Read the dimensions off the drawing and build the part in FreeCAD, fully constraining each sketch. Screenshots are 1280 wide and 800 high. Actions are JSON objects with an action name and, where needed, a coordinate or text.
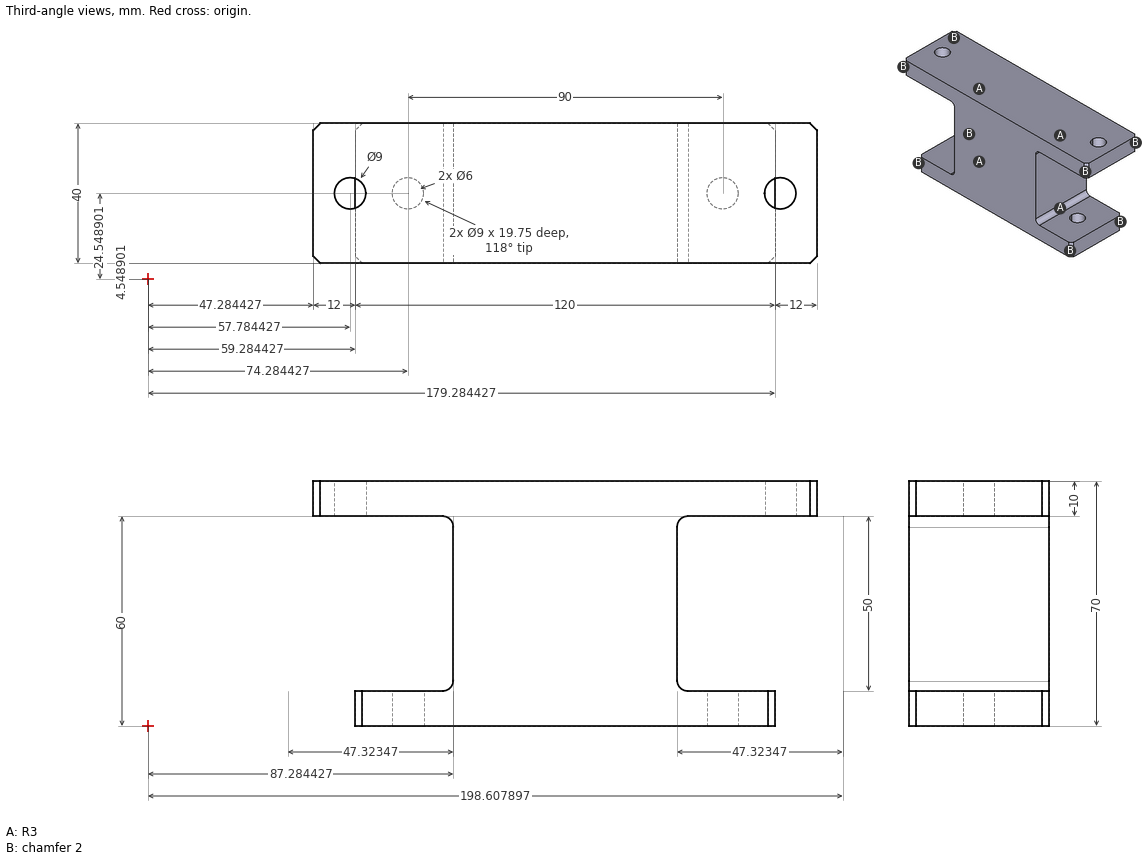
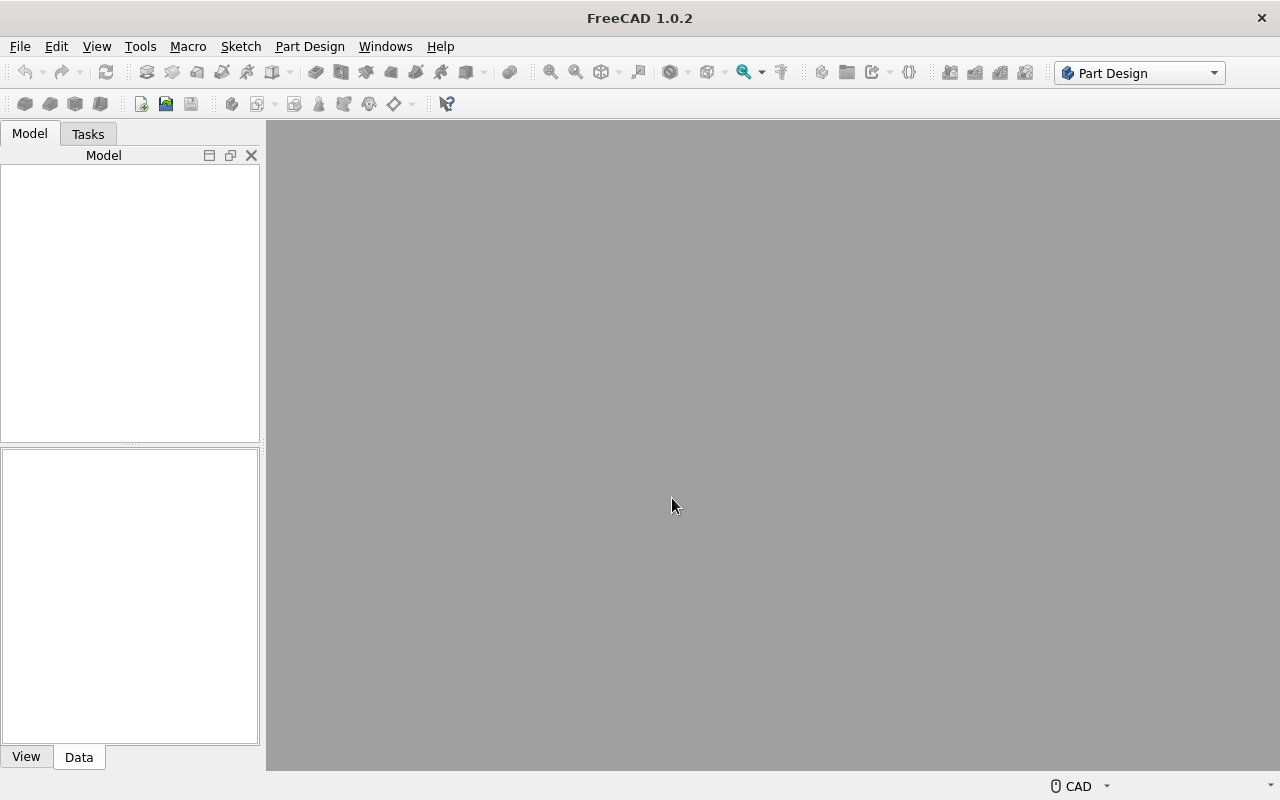
{"action": "key", "text": "ctrl+n"}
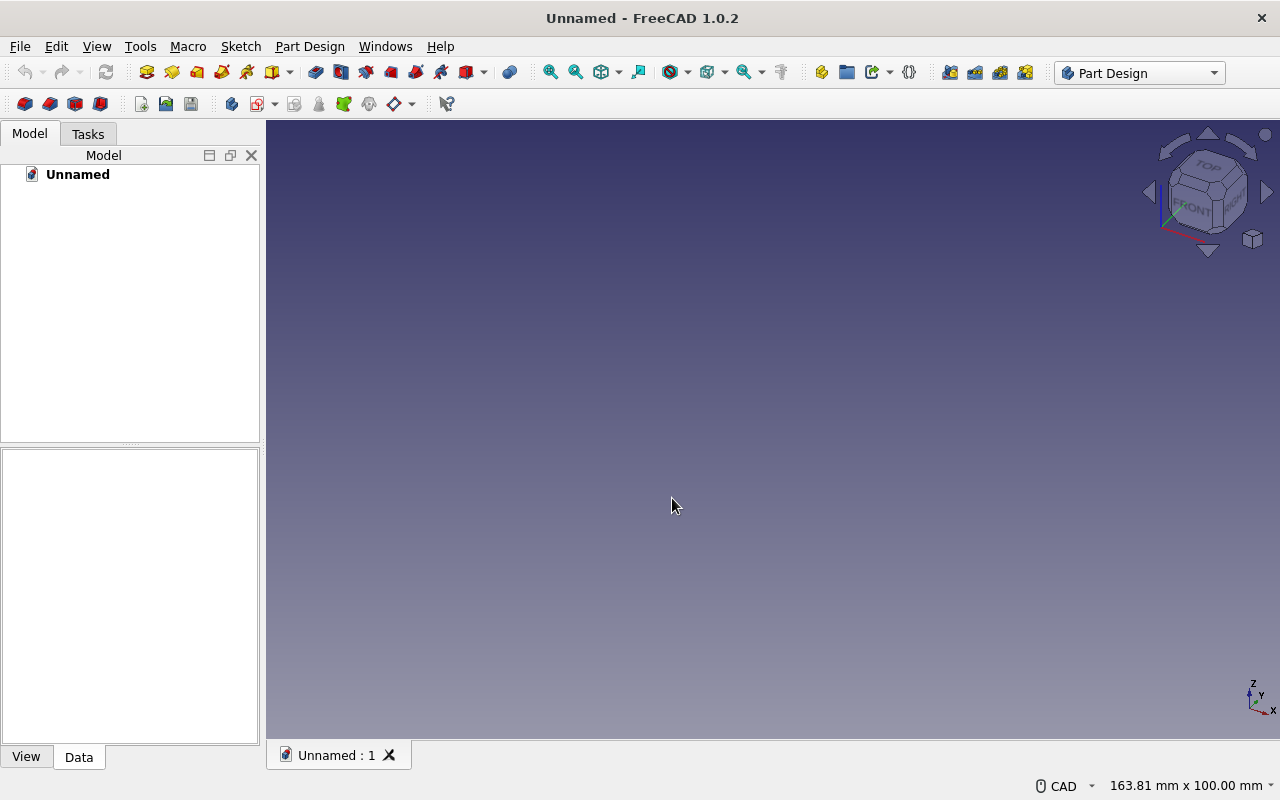
{"action": "left_click", "coordinate": [256, 104]}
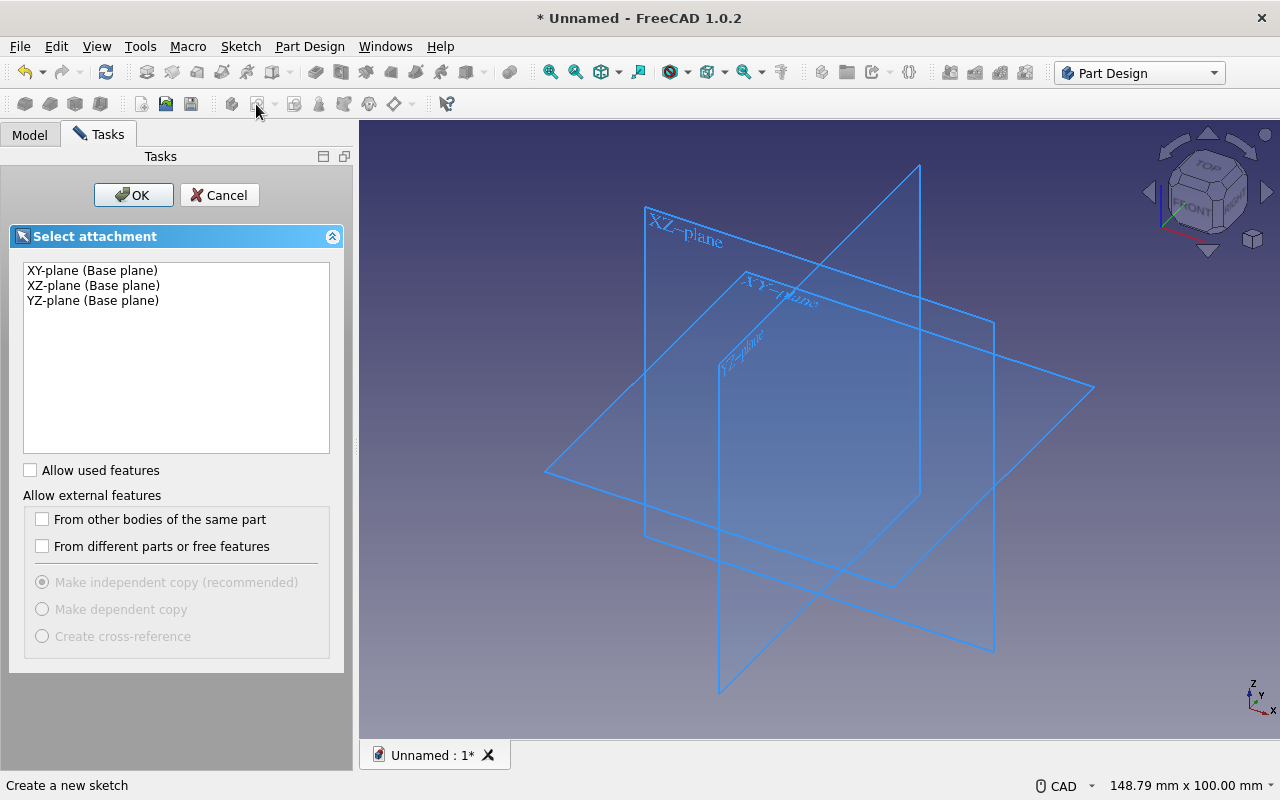
{"action": "left_click", "coordinate": [84, 270]}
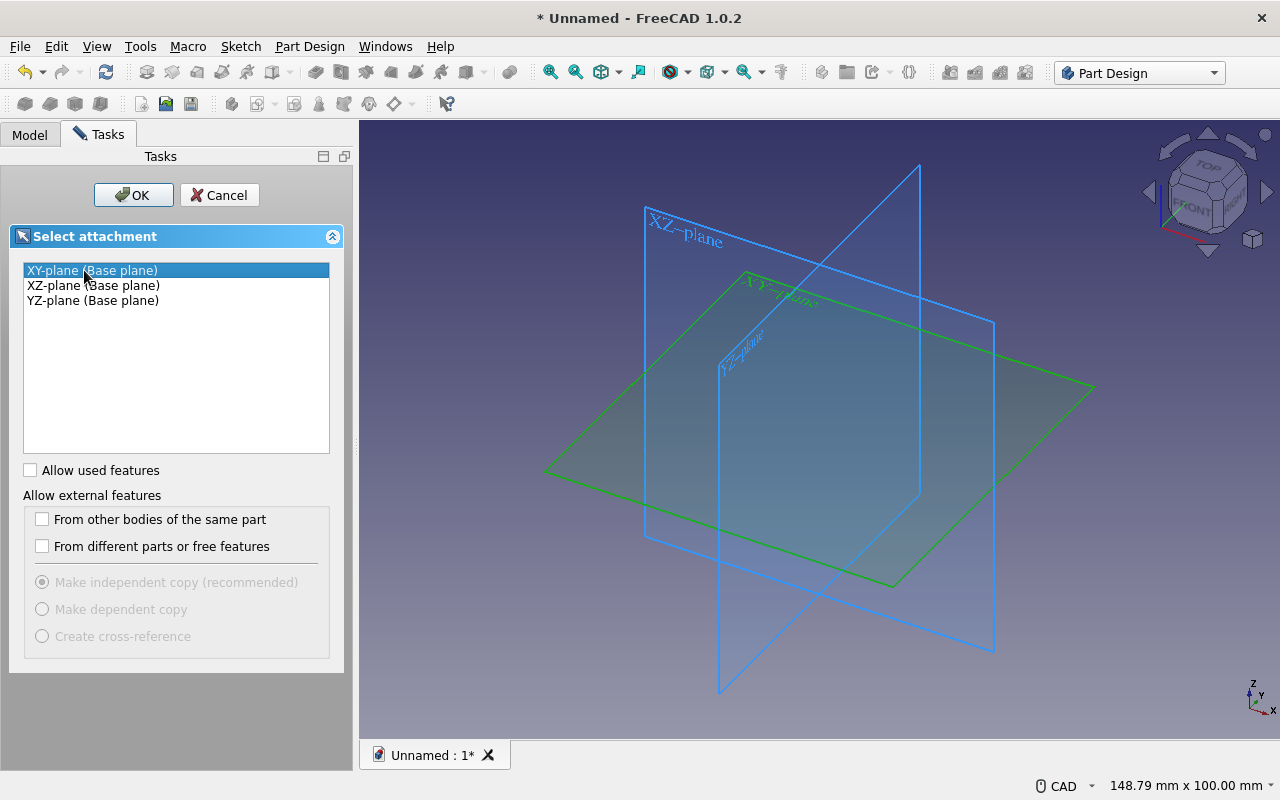
{"action": "left_click", "coordinate": [134, 195]}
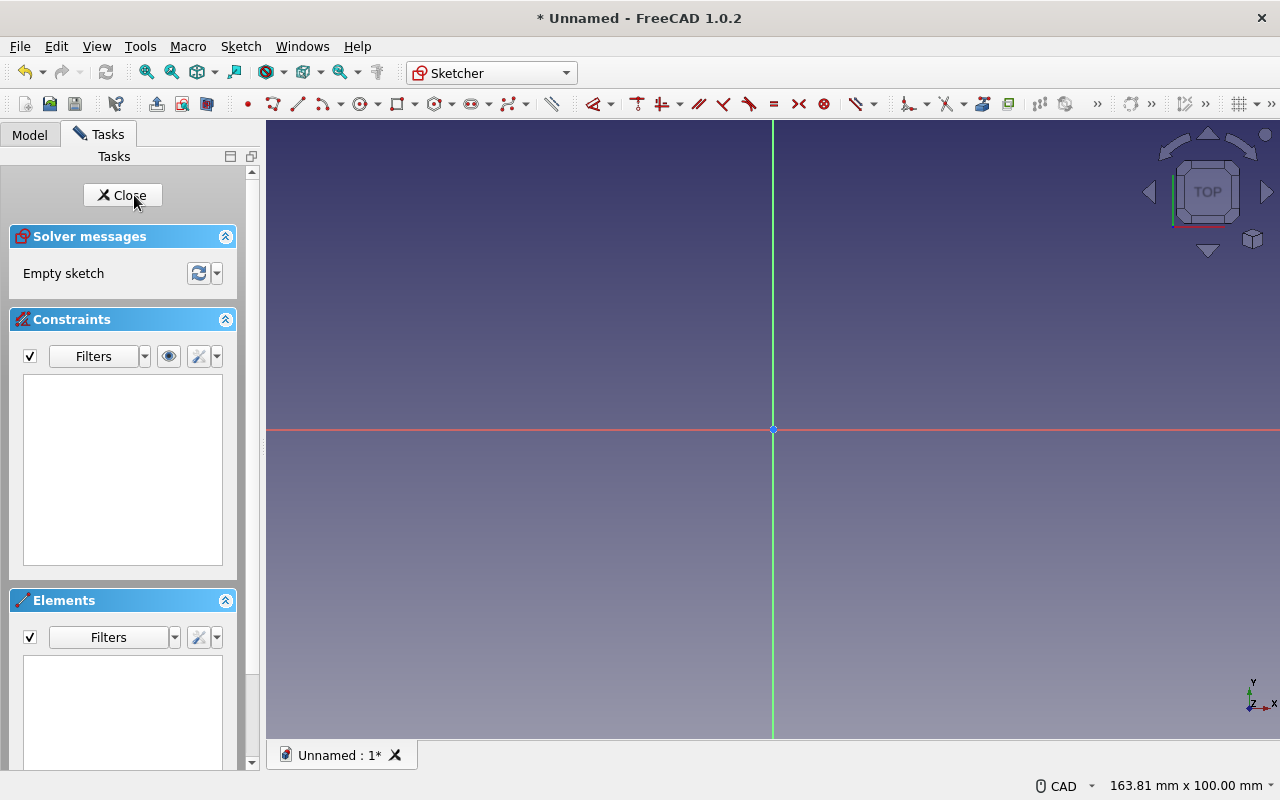
{"action": "scroll", "coordinate": [294, 542], "scroll_direction": "down", "scroll_amount": 4}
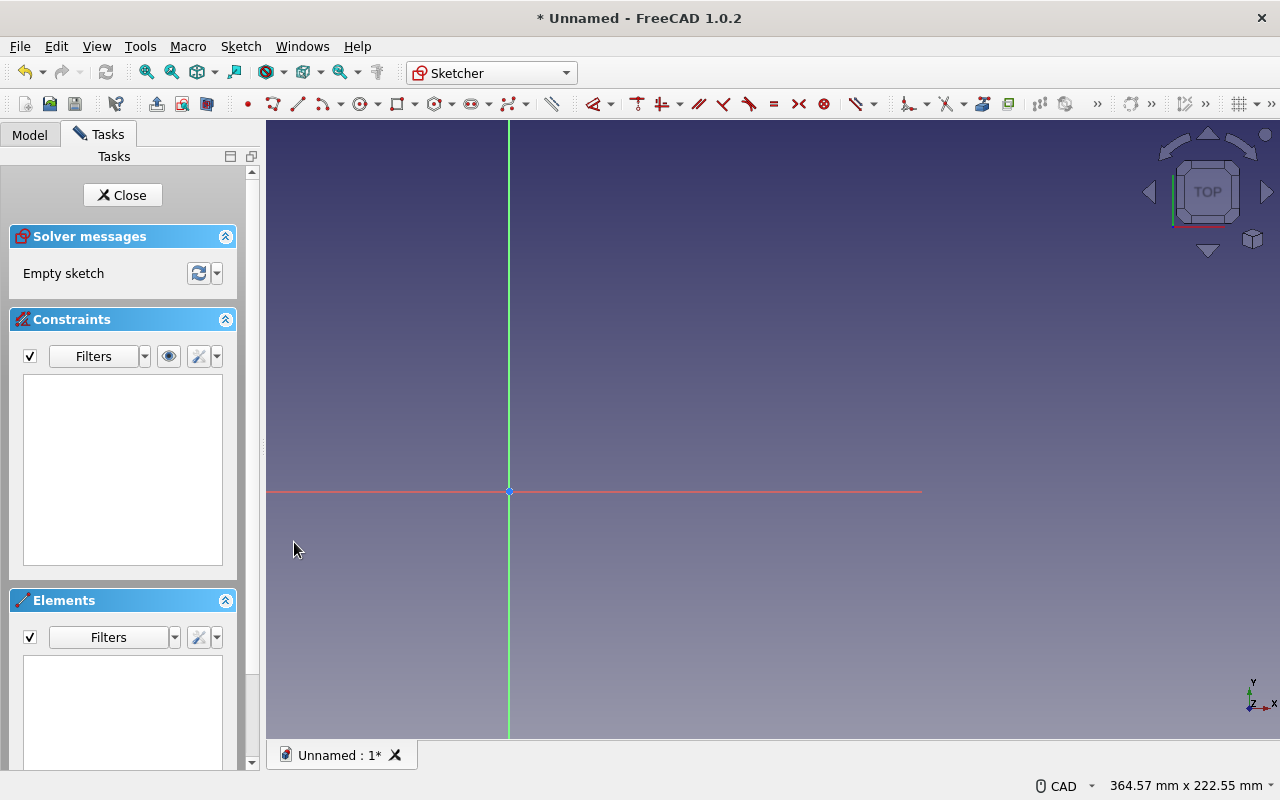
{"action": "key", "text": "g r"}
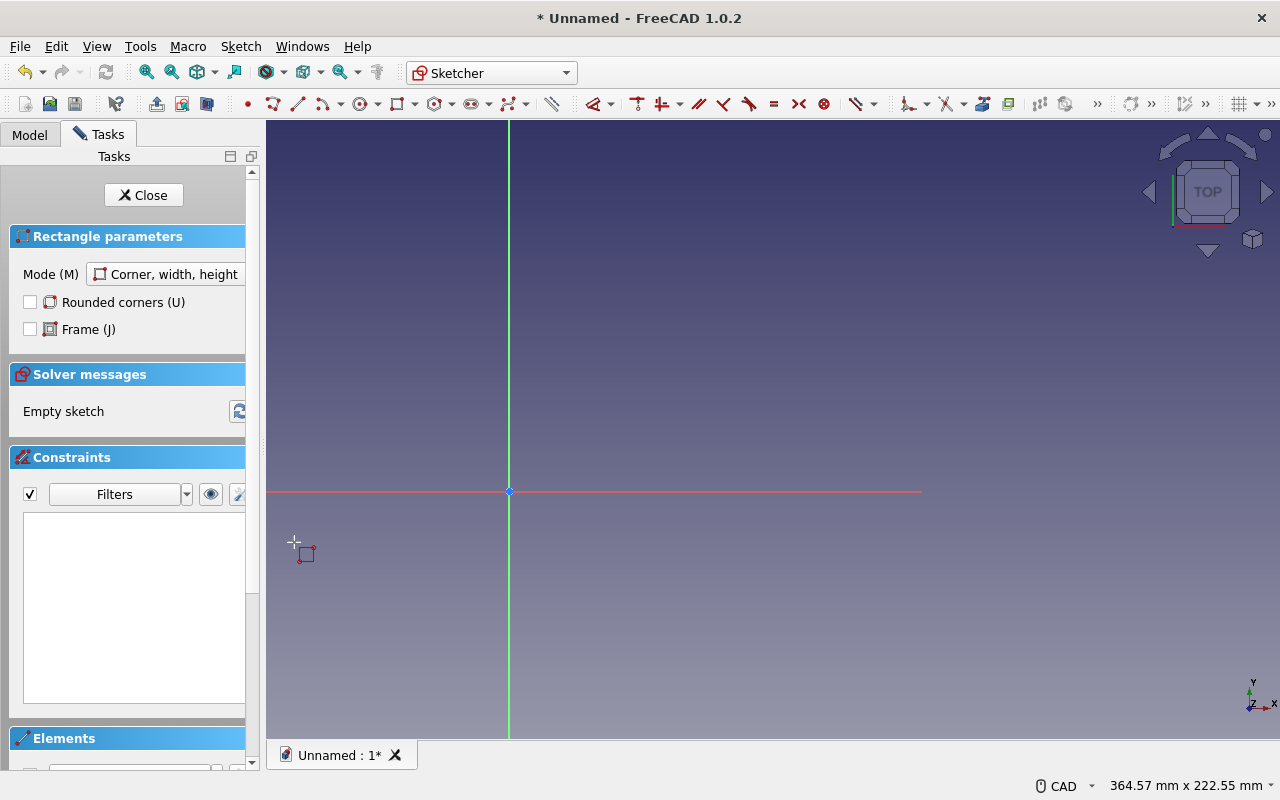
{"action": "left_click", "coordinate": [674, 368]}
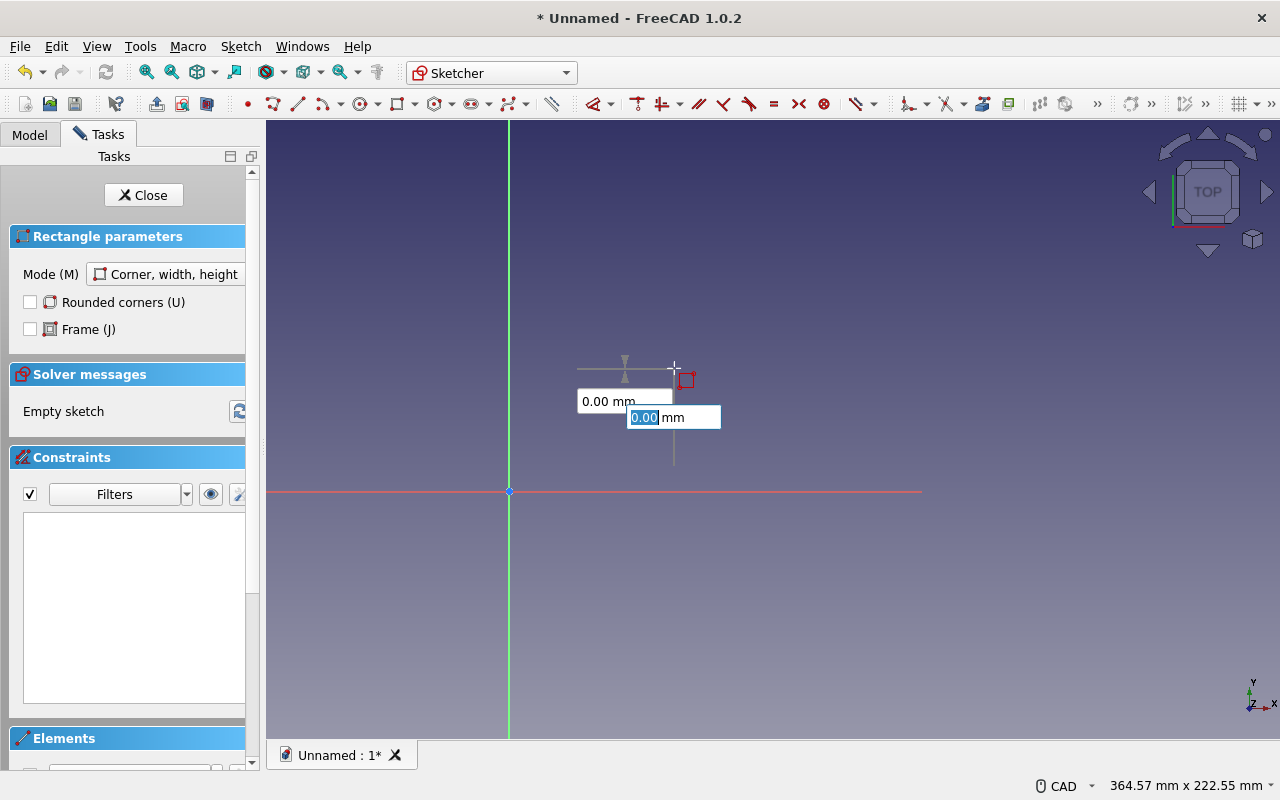
{"action": "scroll", "coordinate": [1008, 479], "scroll_direction": "up", "scroll_amount": 2}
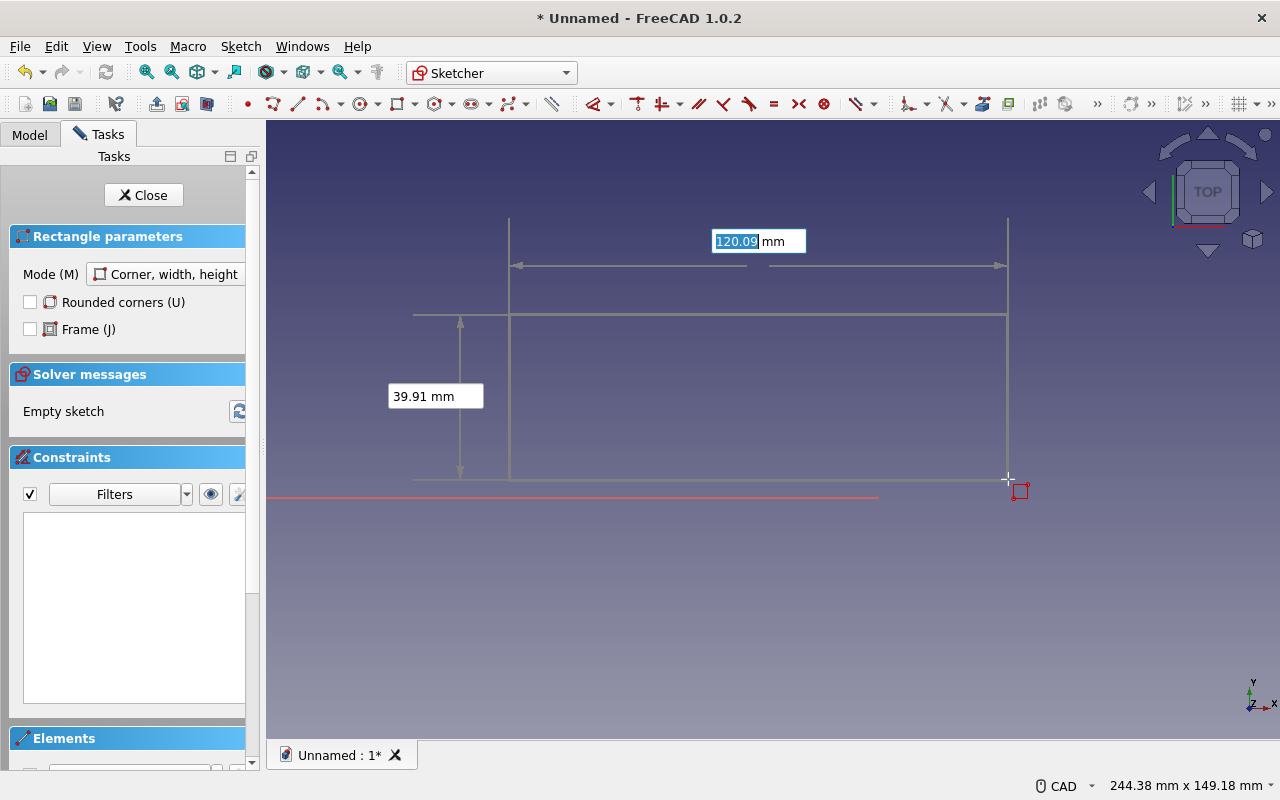
{"action": "left_click", "coordinate": [1007, 479]}
{"action": "key", "text": "Escape"}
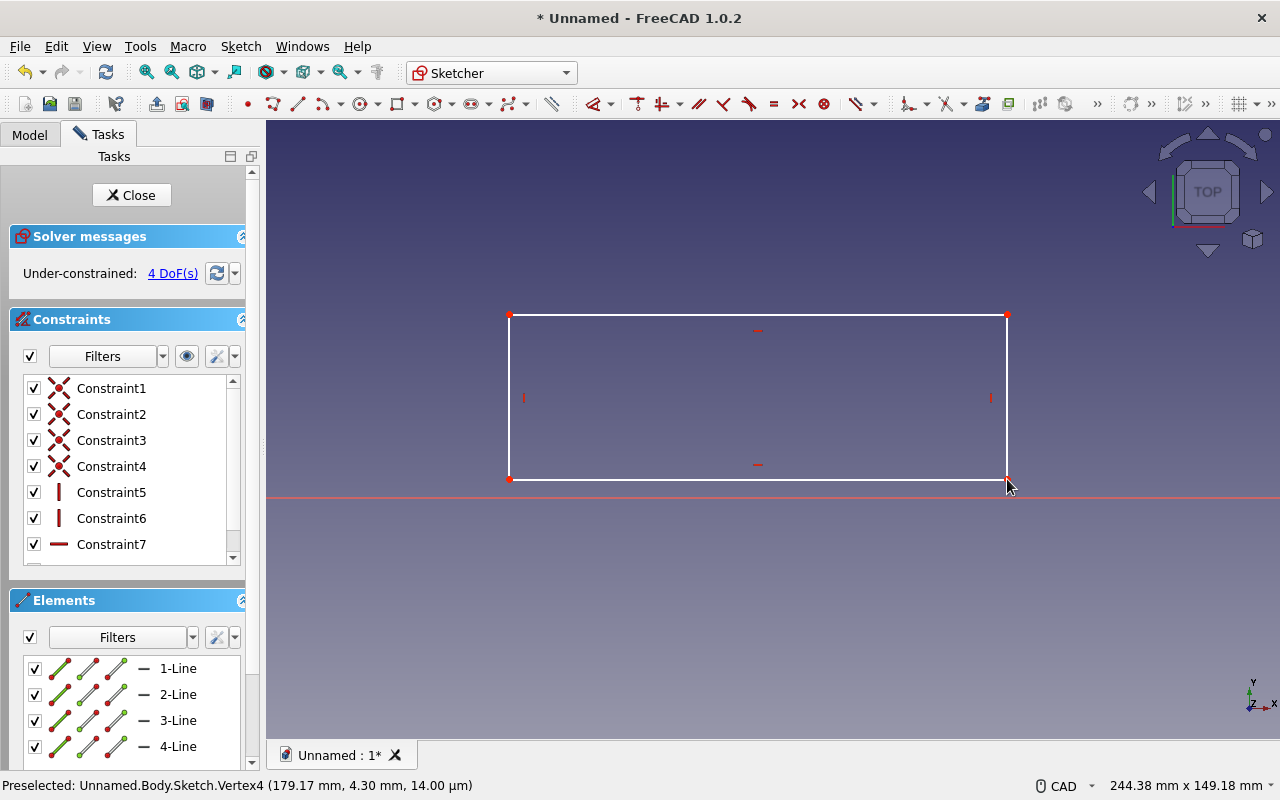
{"action": "left_click", "coordinate": [509, 364]}